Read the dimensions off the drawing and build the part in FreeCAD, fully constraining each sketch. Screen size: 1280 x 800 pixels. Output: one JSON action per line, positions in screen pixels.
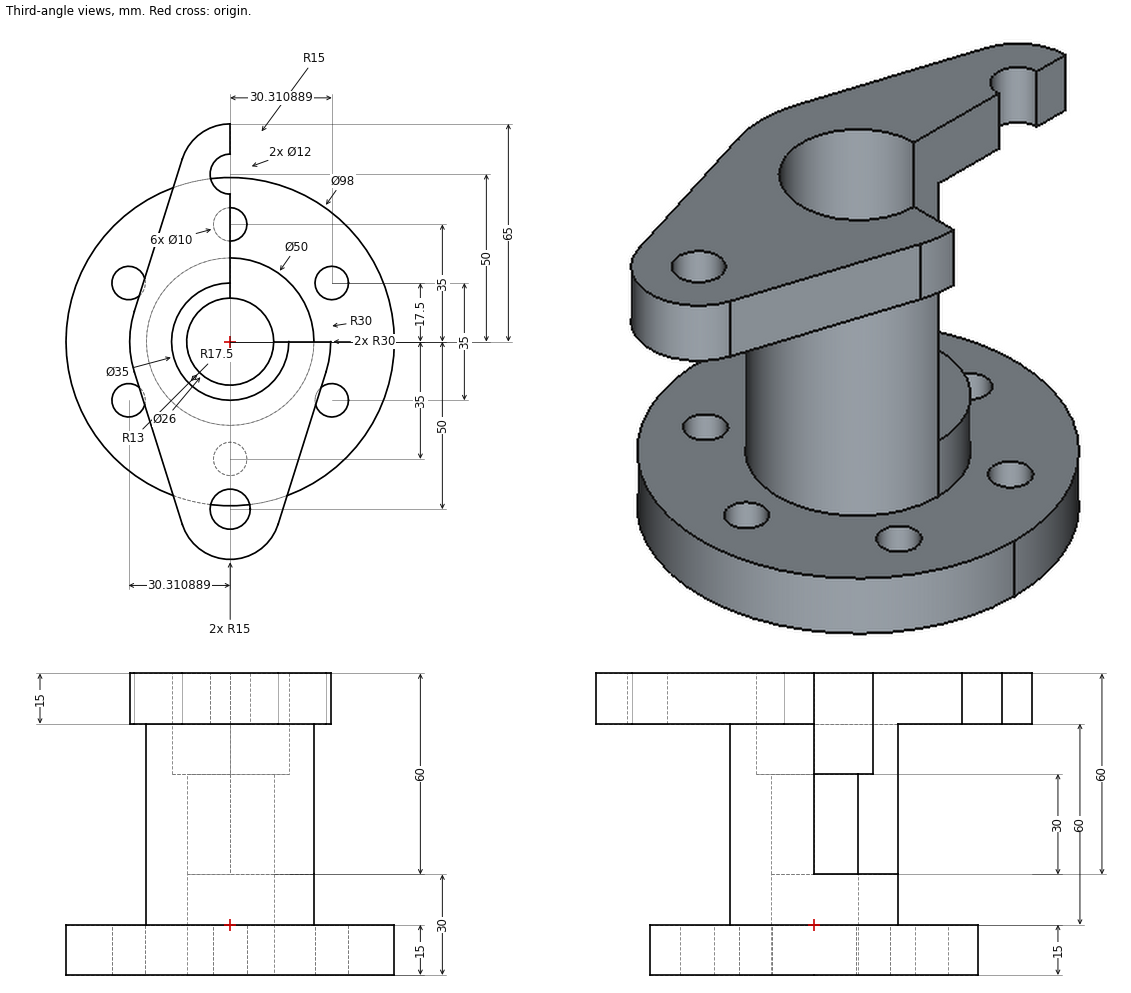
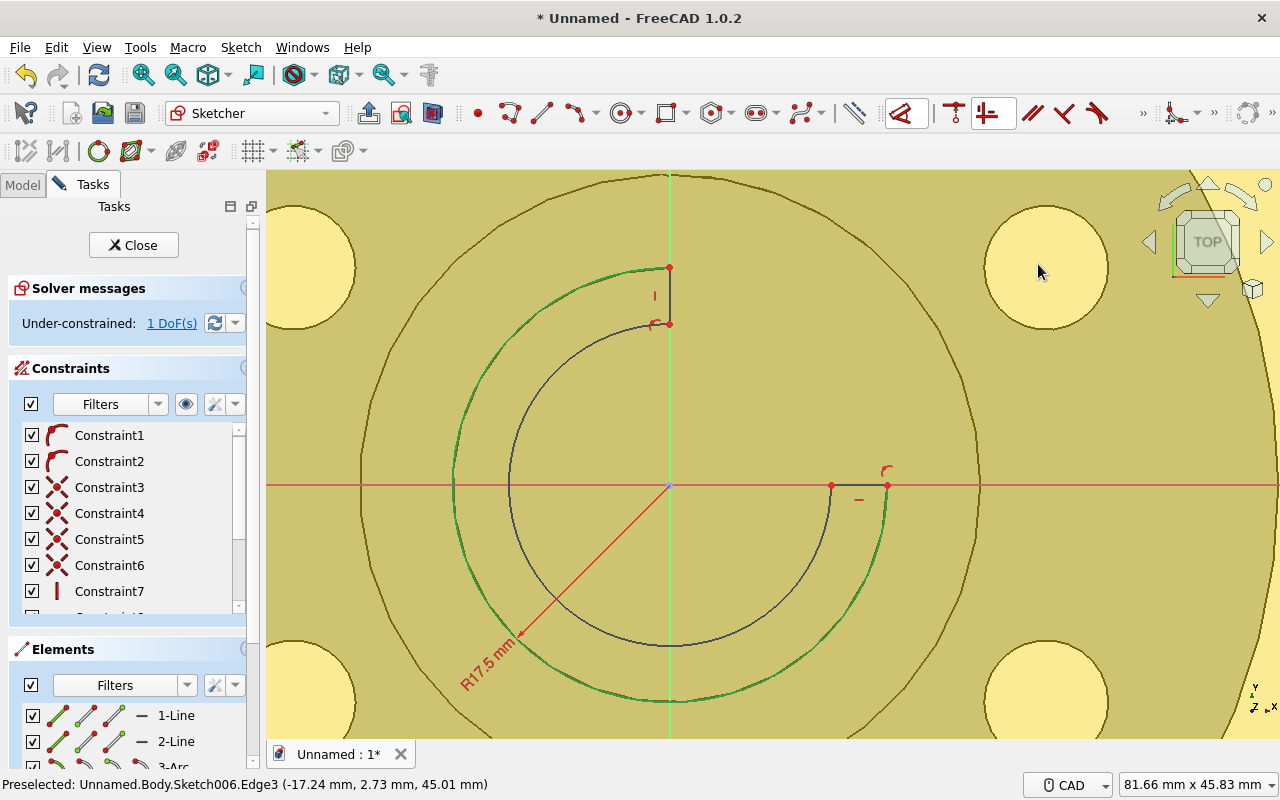
{"action": "left_click", "coordinate": [511, 460]}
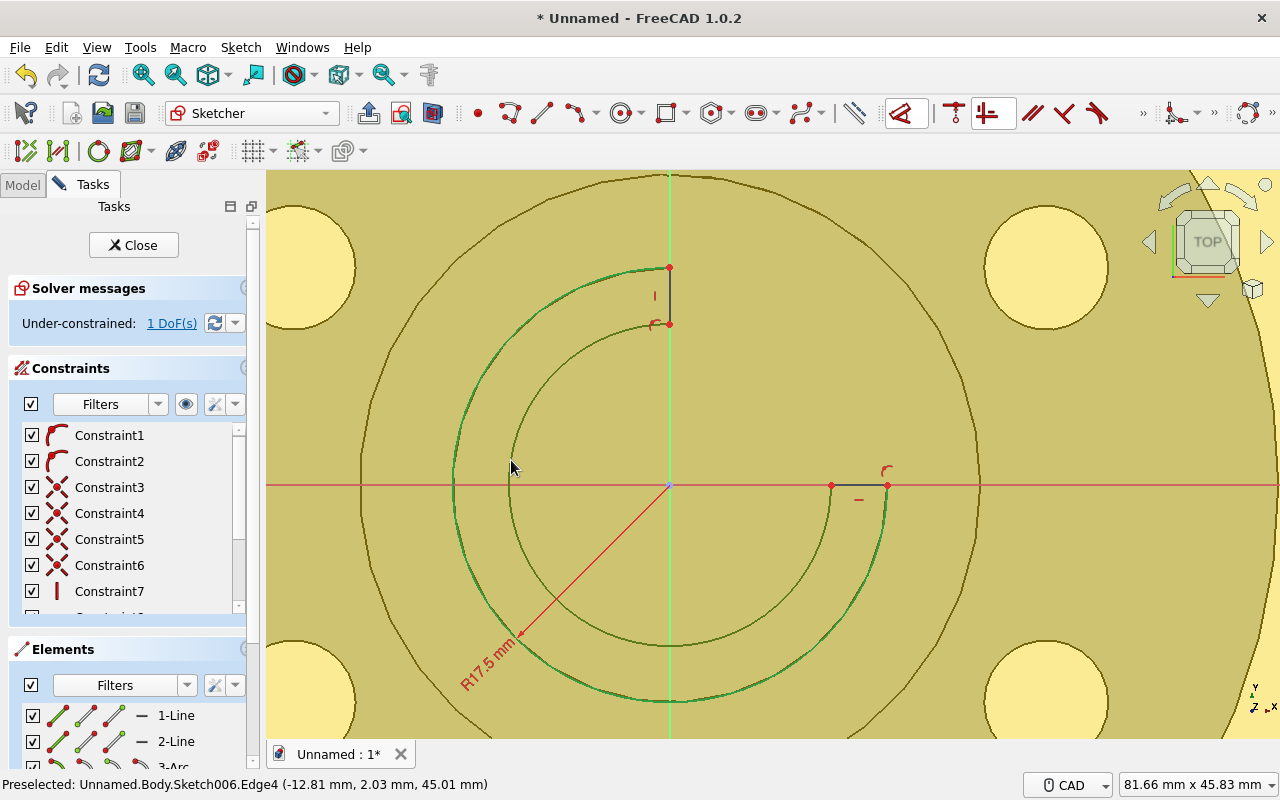
{"action": "key", "text": "k r"}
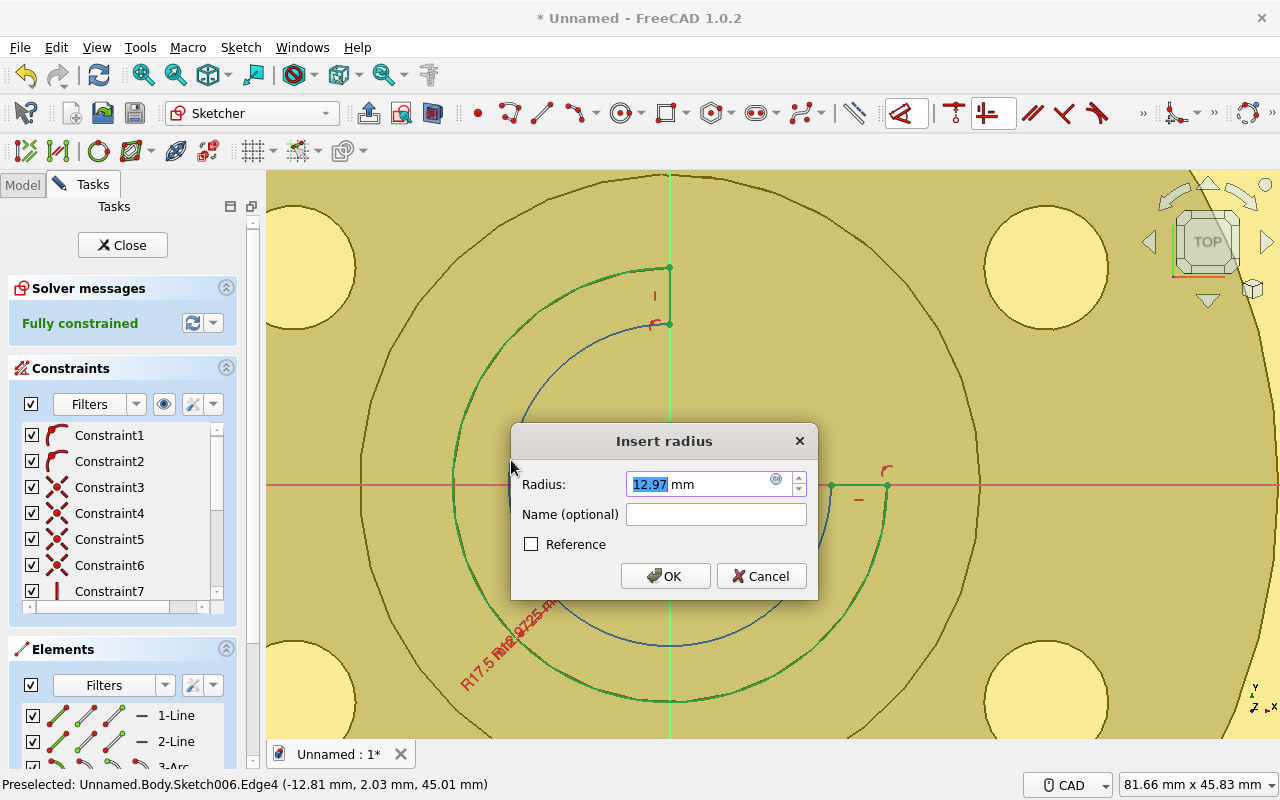
{"action": "type", "text": "13"}
{"action": "key", "text": "Return"}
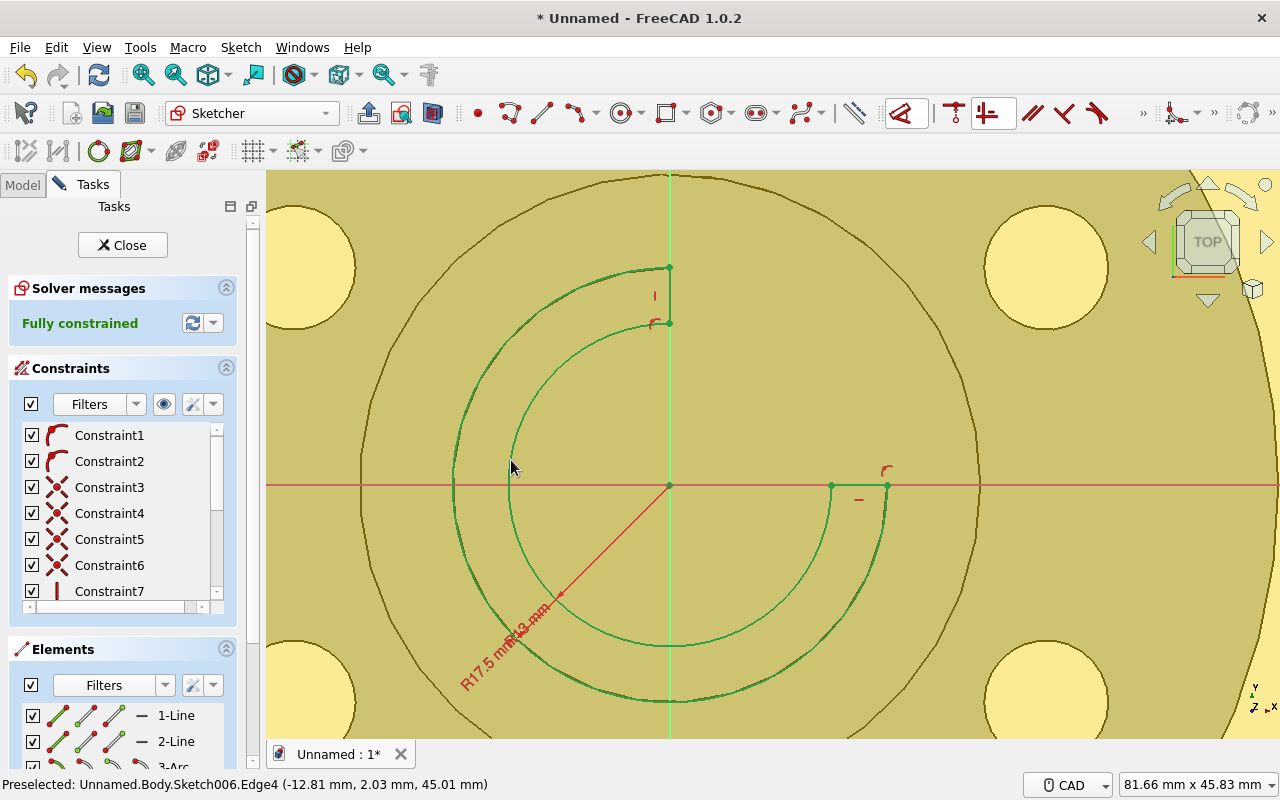
{"action": "left_click", "coordinate": [123, 245]}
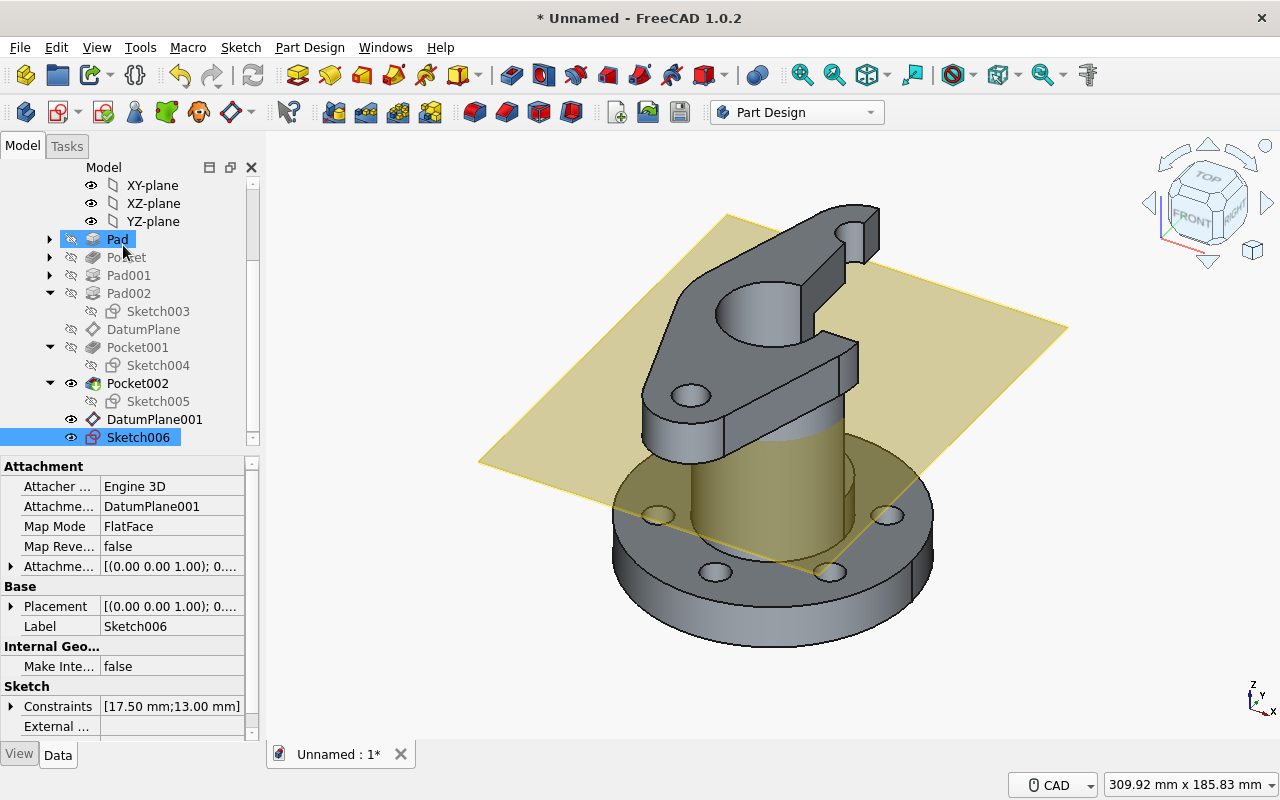
{"action": "left_click", "coordinate": [298, 76]}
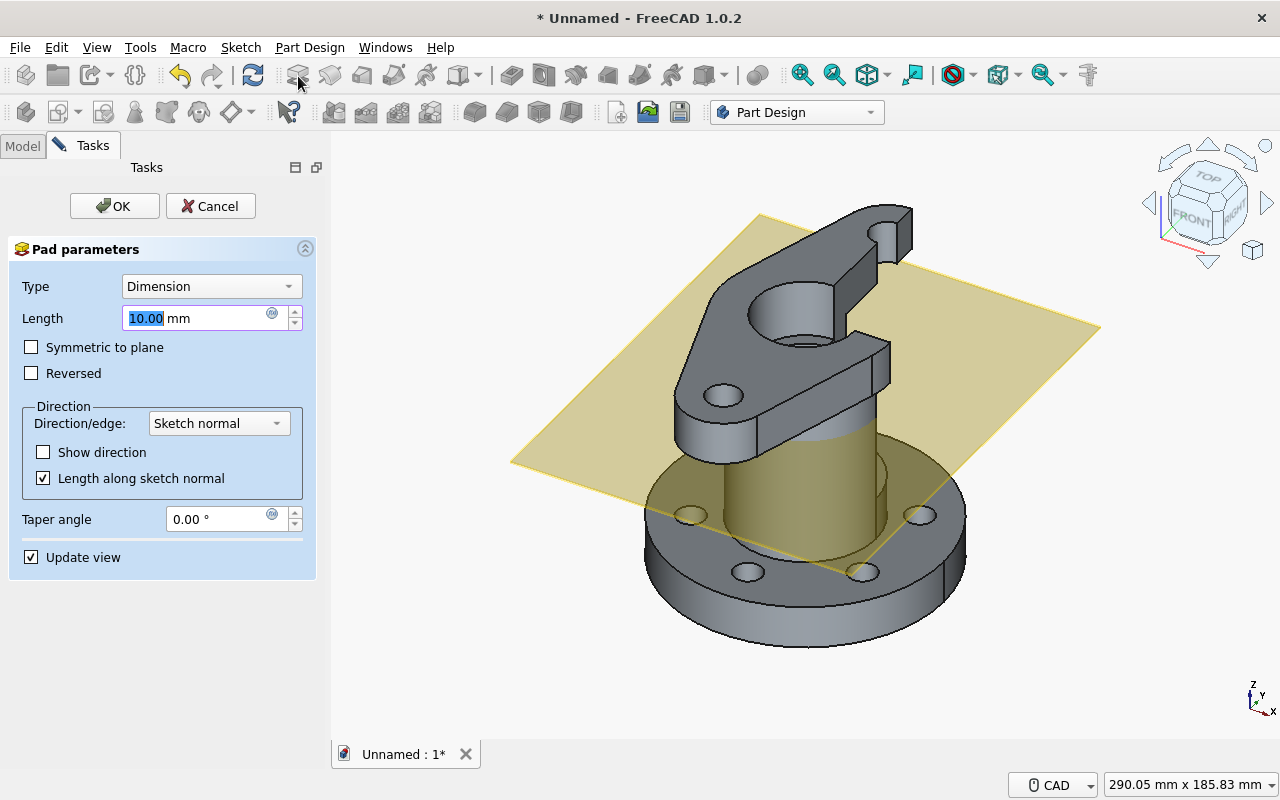
{"action": "type", "text": "30"}
{"action": "key", "text": "Tab"}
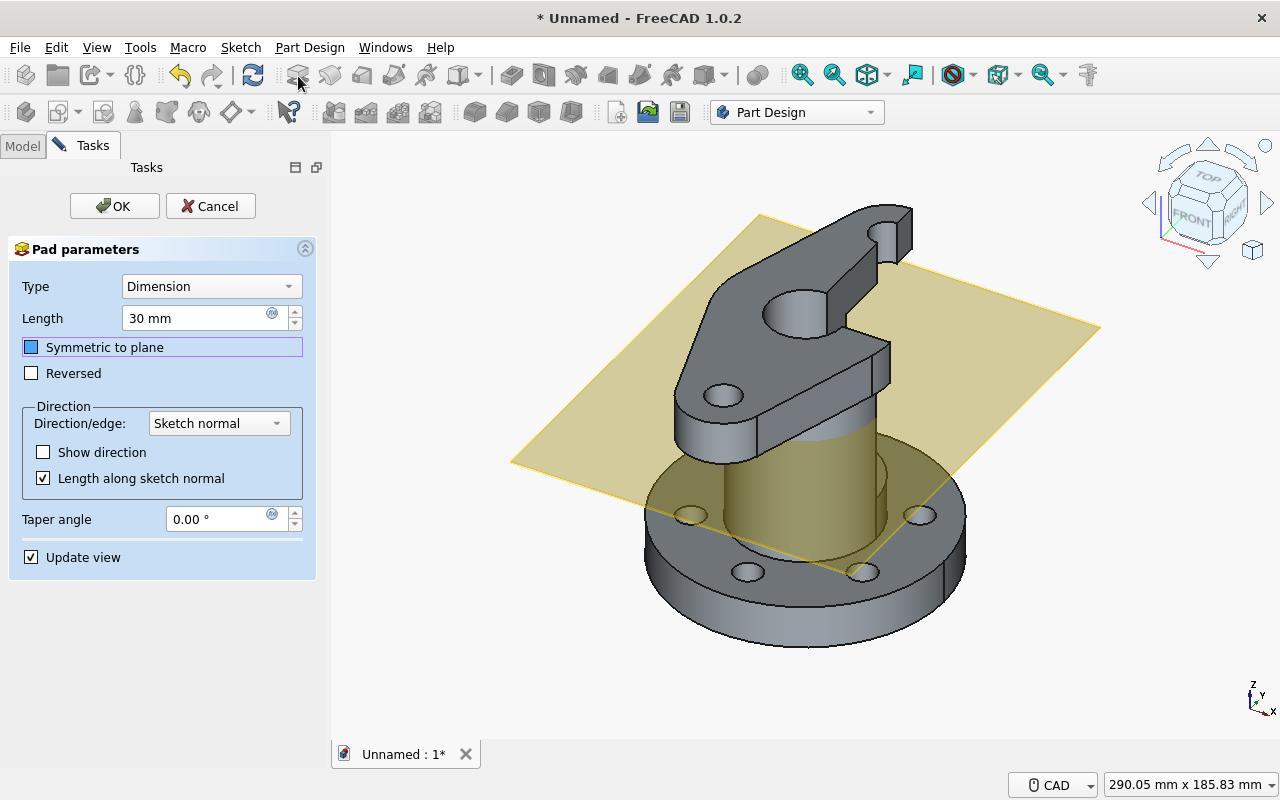
{"action": "left_click", "coordinate": [30, 373]}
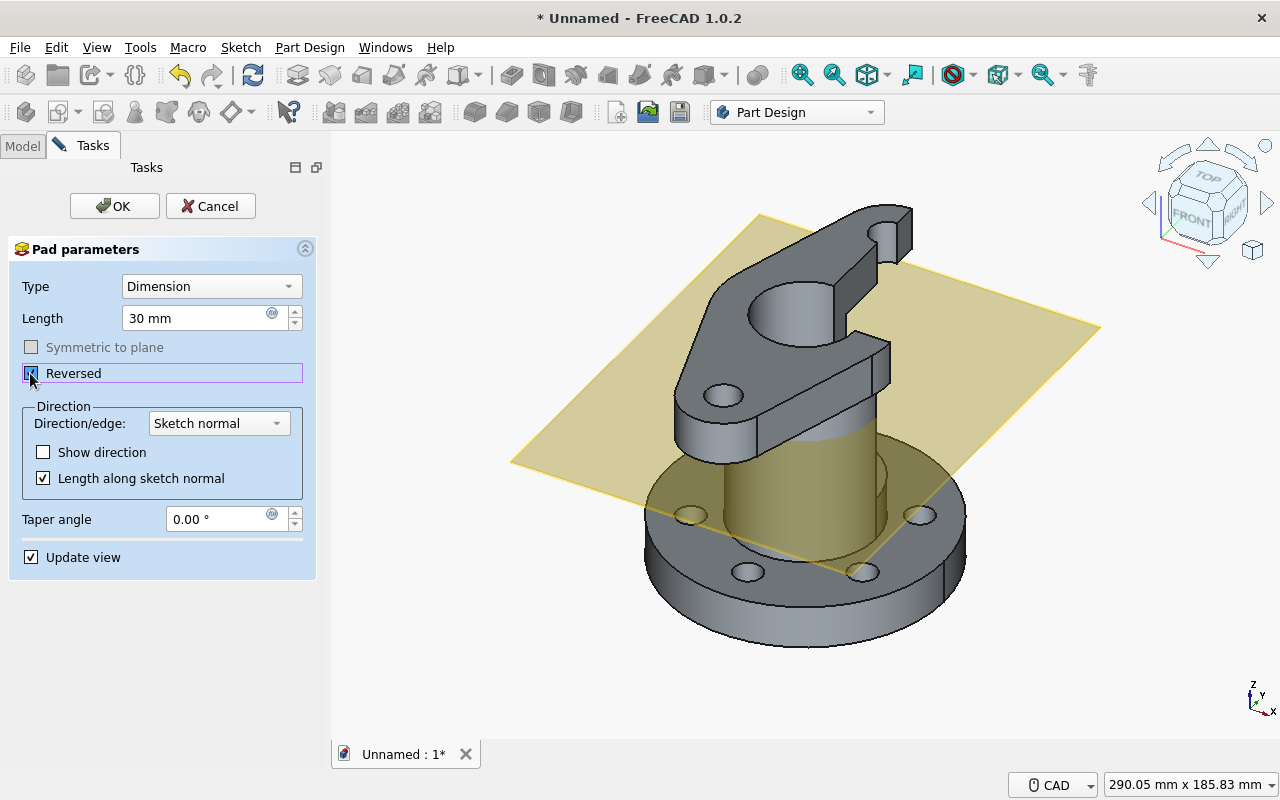
{"action": "left_click", "coordinate": [115, 206]}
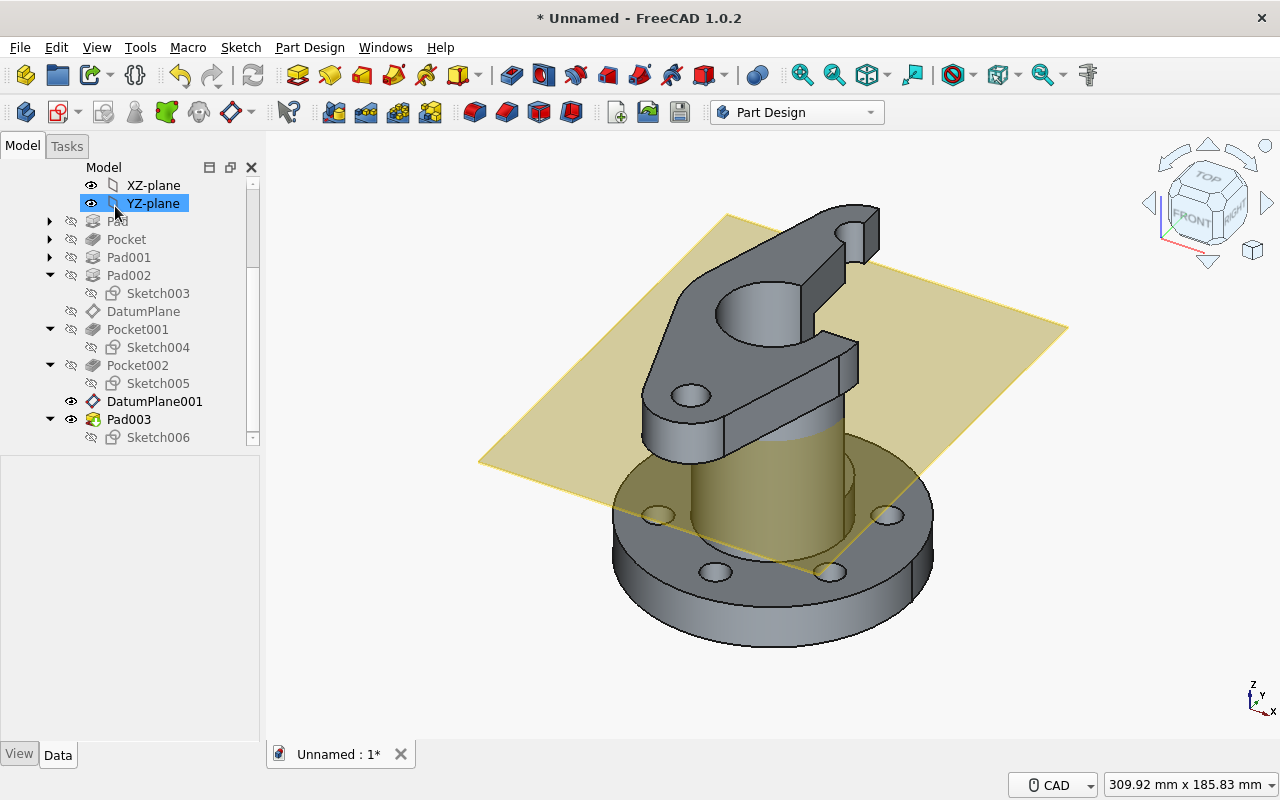
{"action": "left_click", "coordinate": [116, 401]}
{"action": "key", "text": "space"}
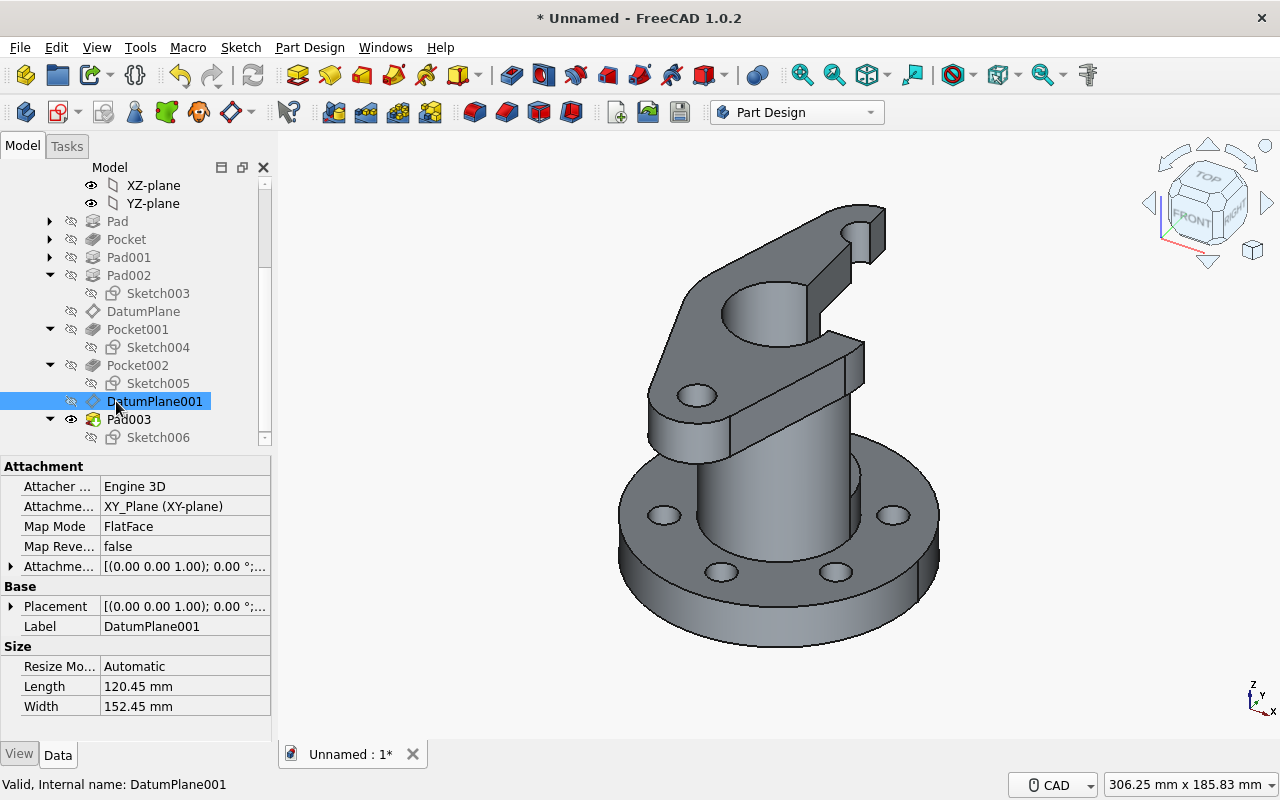
{"action": "key", "text": "0"}